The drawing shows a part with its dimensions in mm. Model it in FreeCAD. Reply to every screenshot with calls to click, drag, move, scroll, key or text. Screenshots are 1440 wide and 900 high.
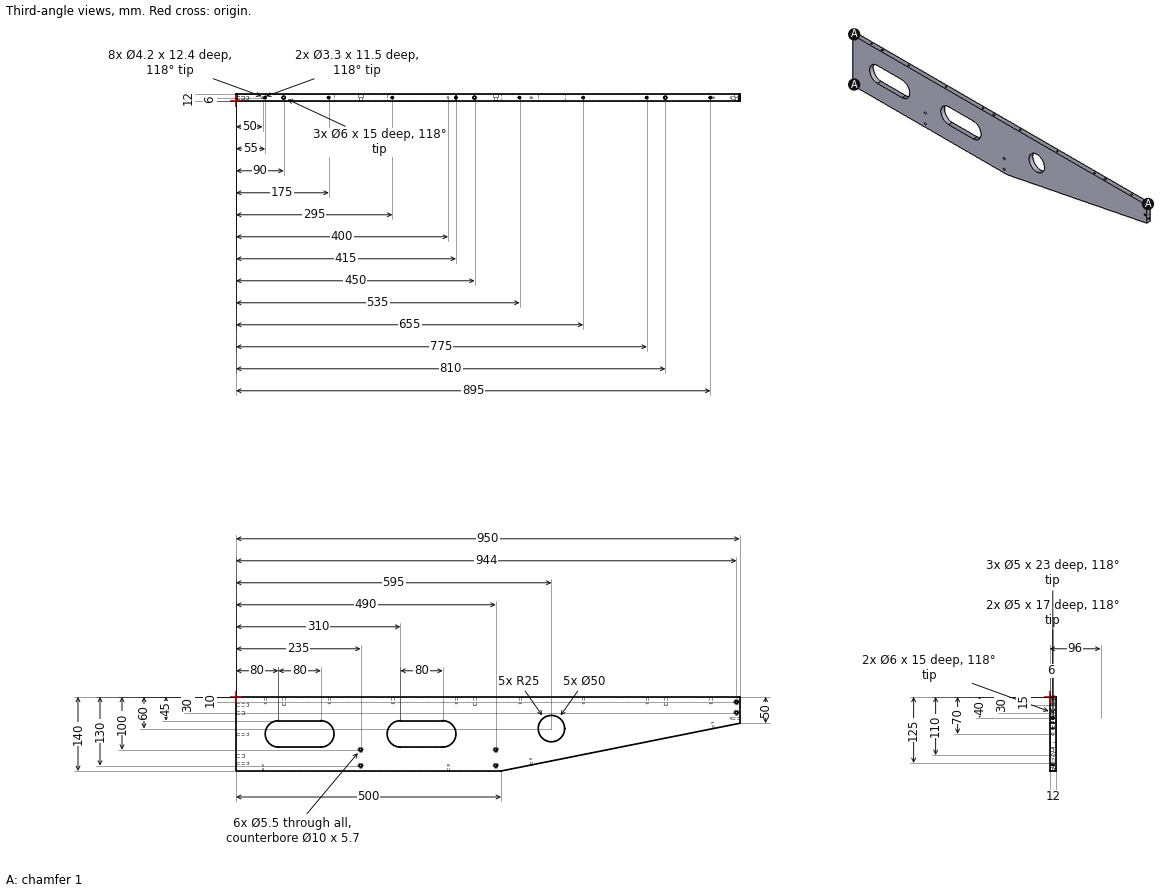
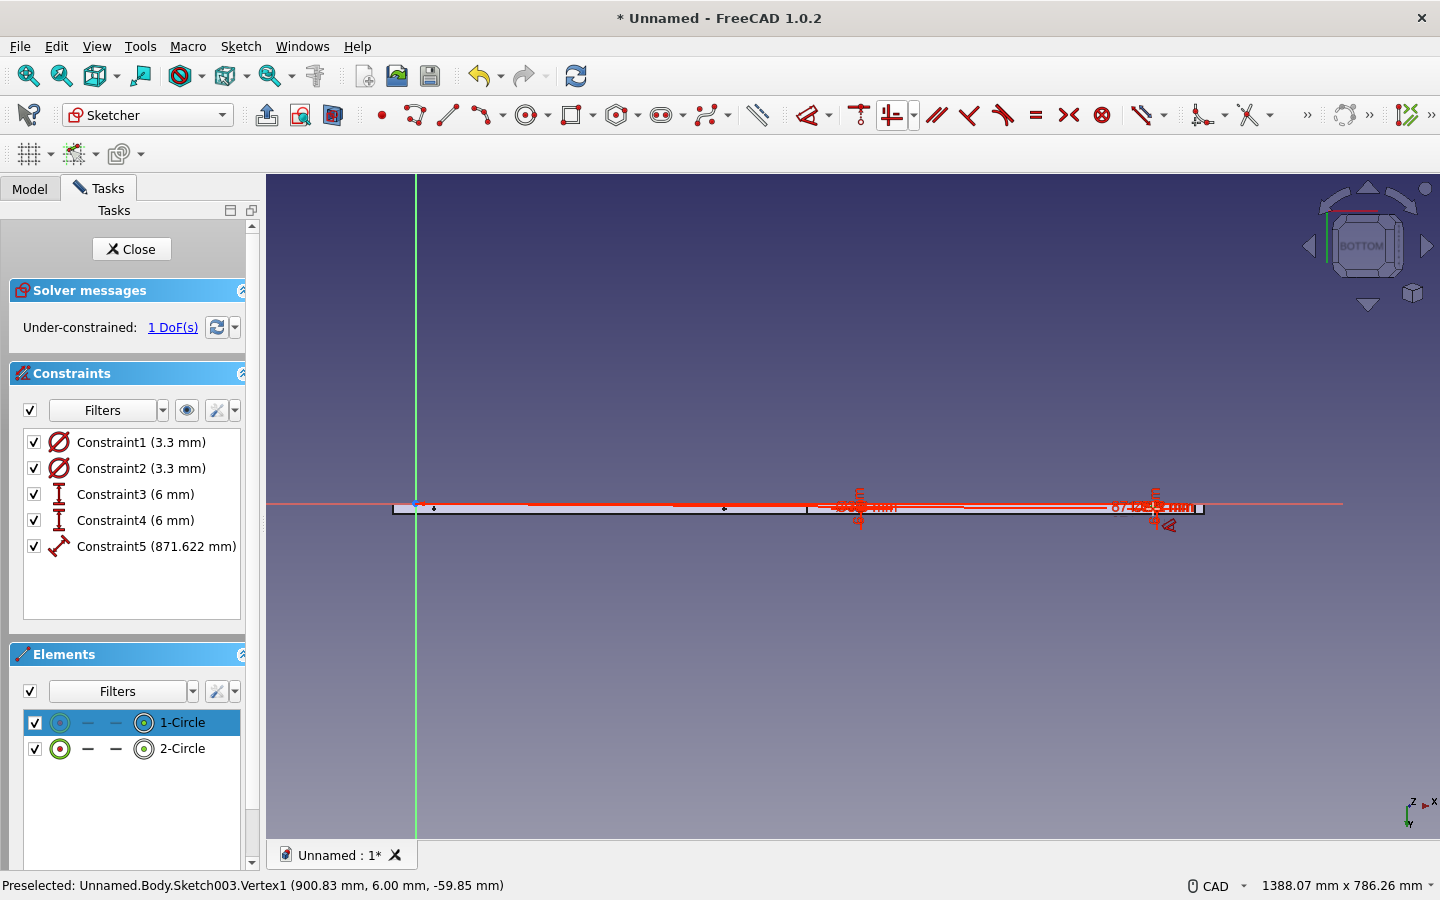
click(857, 509)
click(1005, 543)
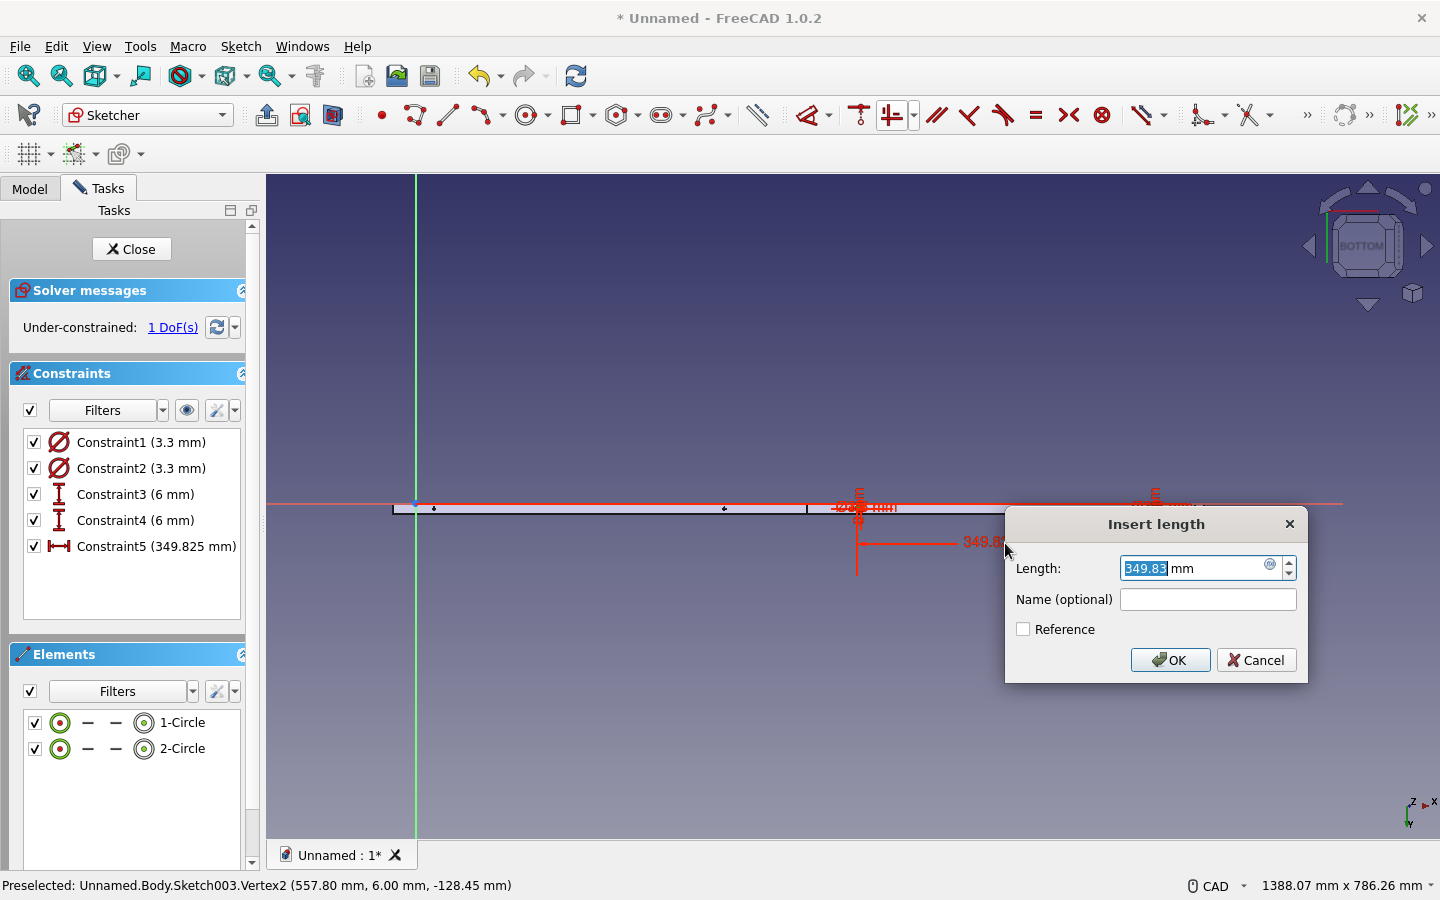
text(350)
key(Return)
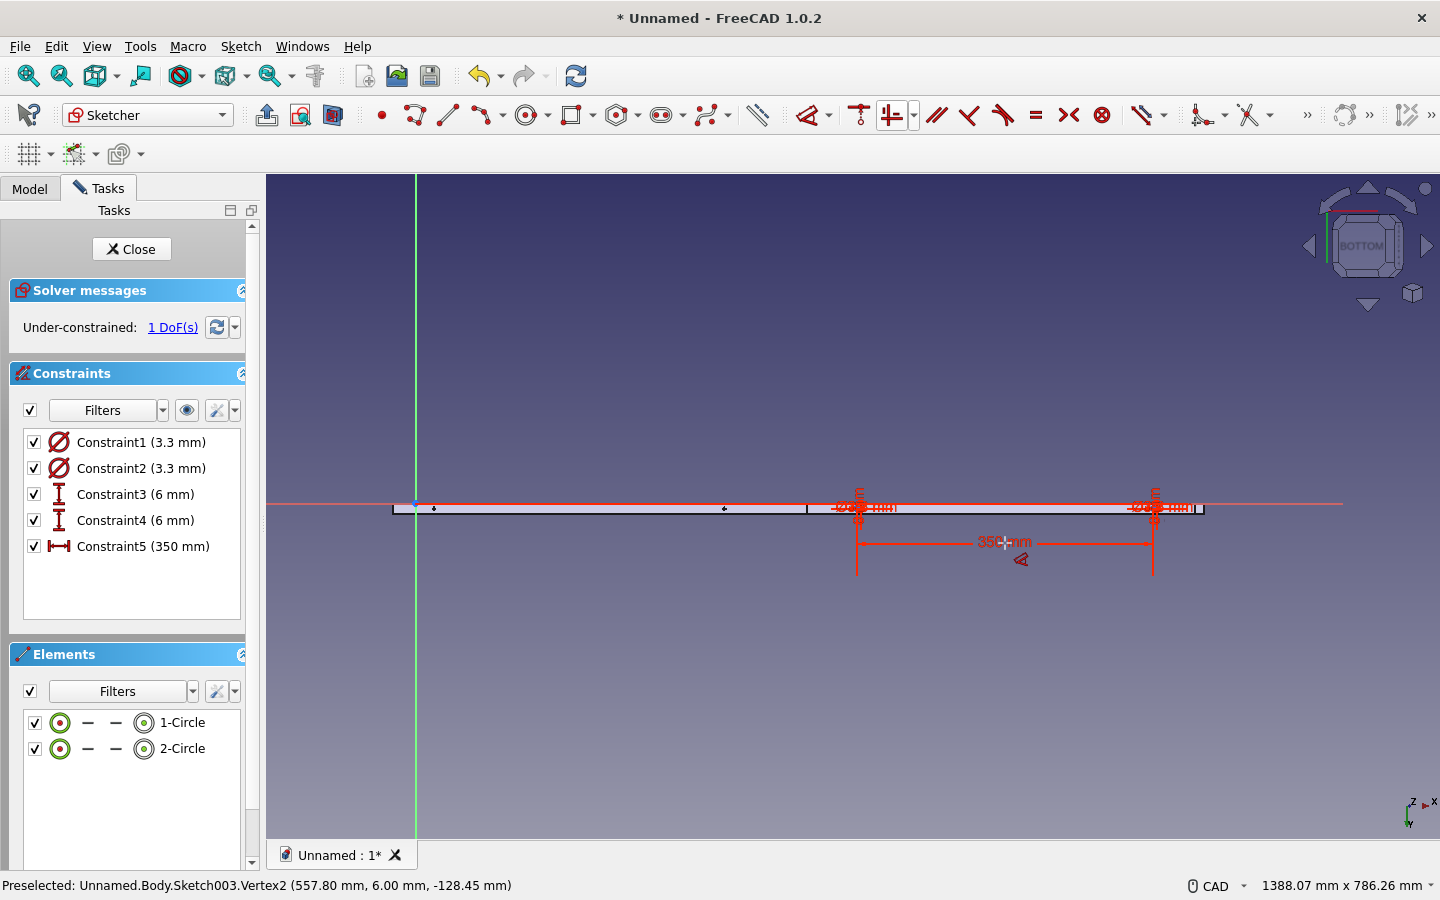
click(1153, 509)
click(784, 470)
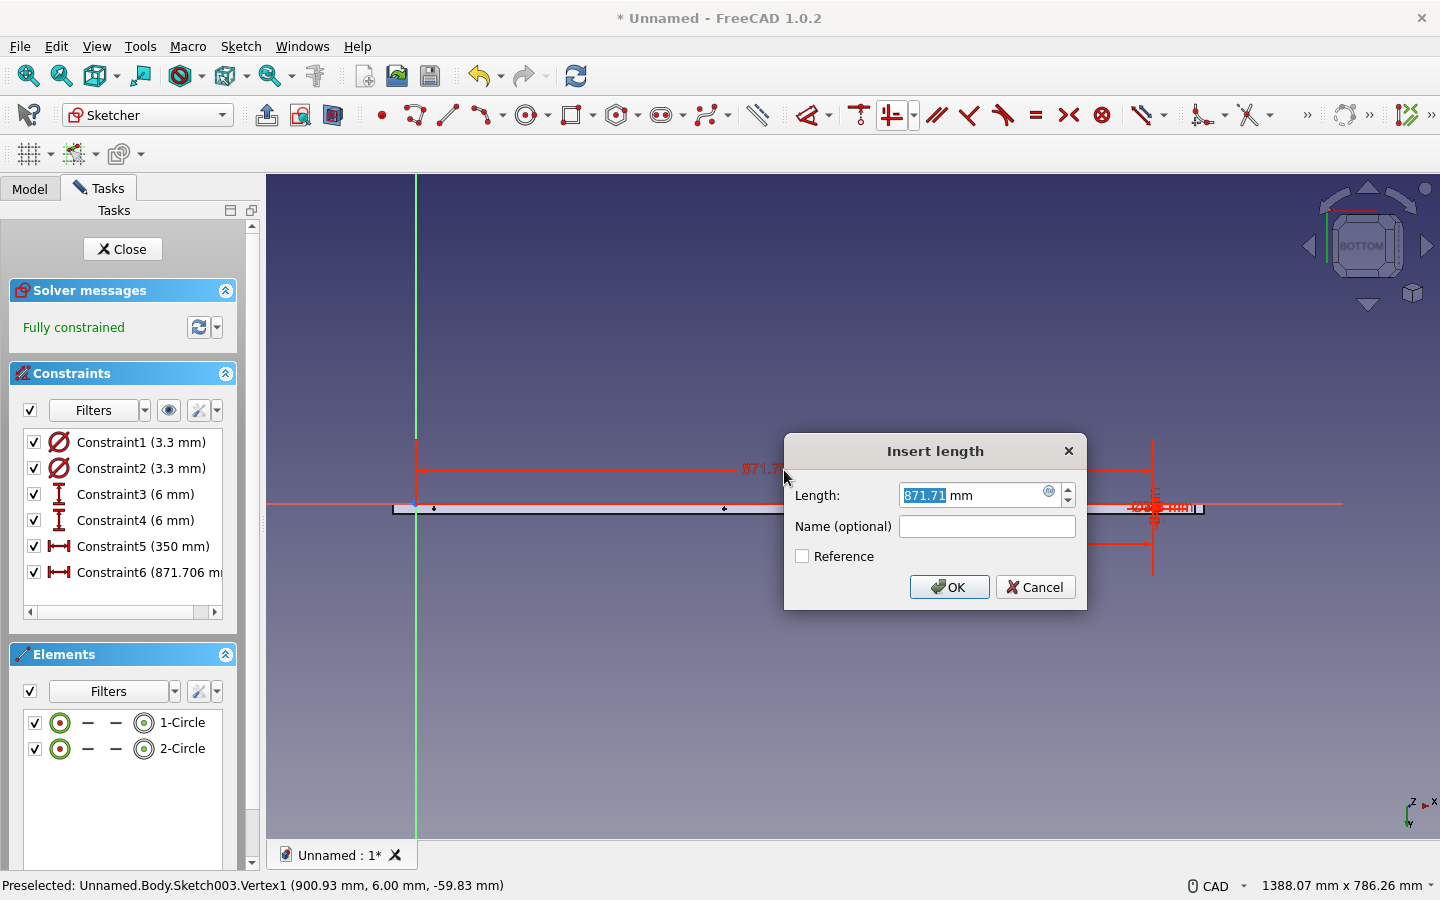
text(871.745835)
key(Return)
key(Escape)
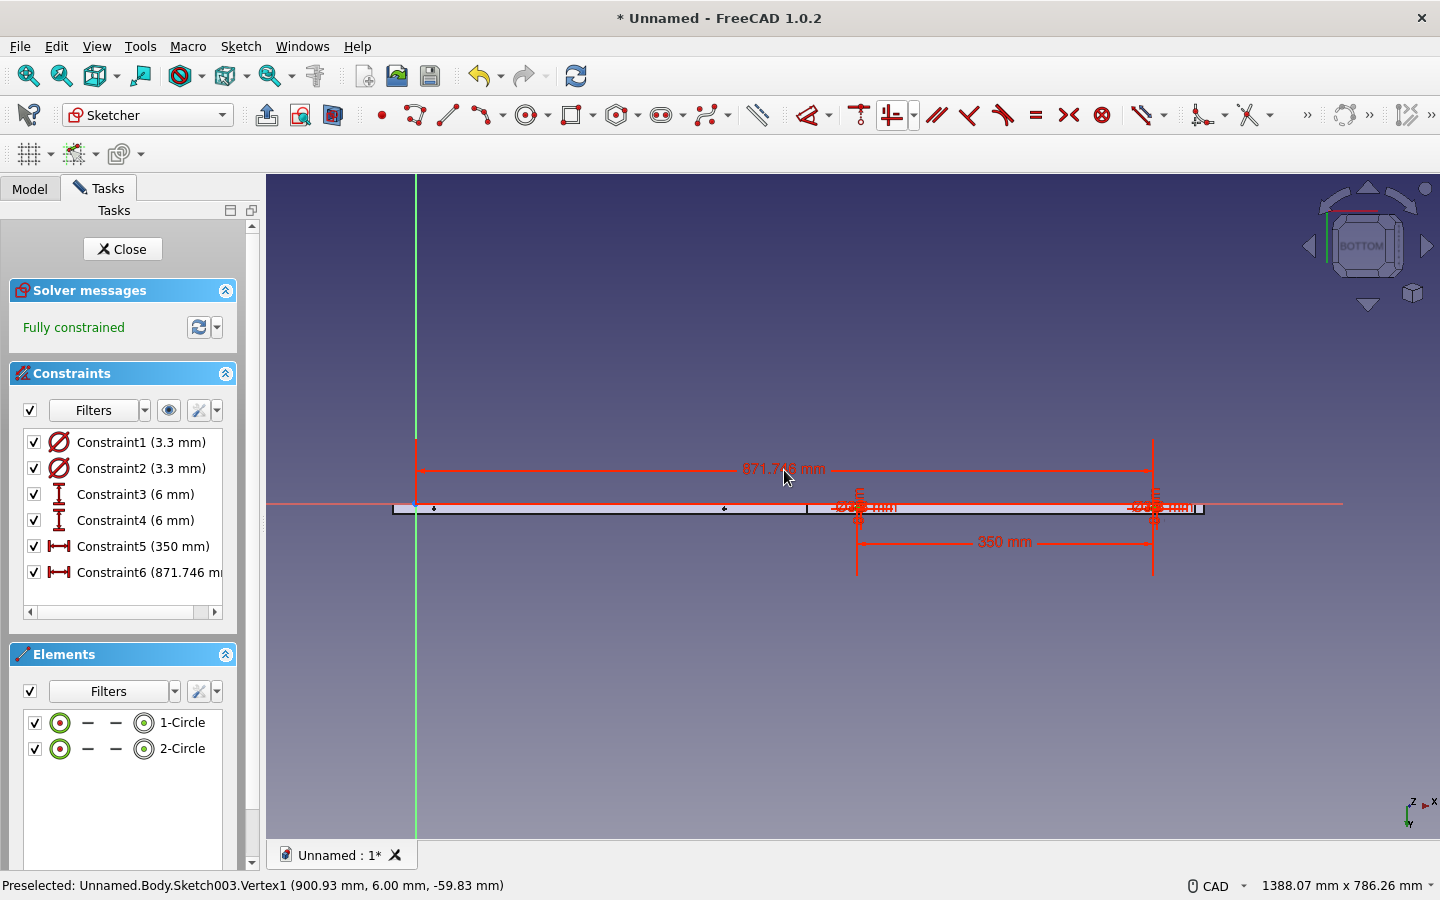
click(123, 249)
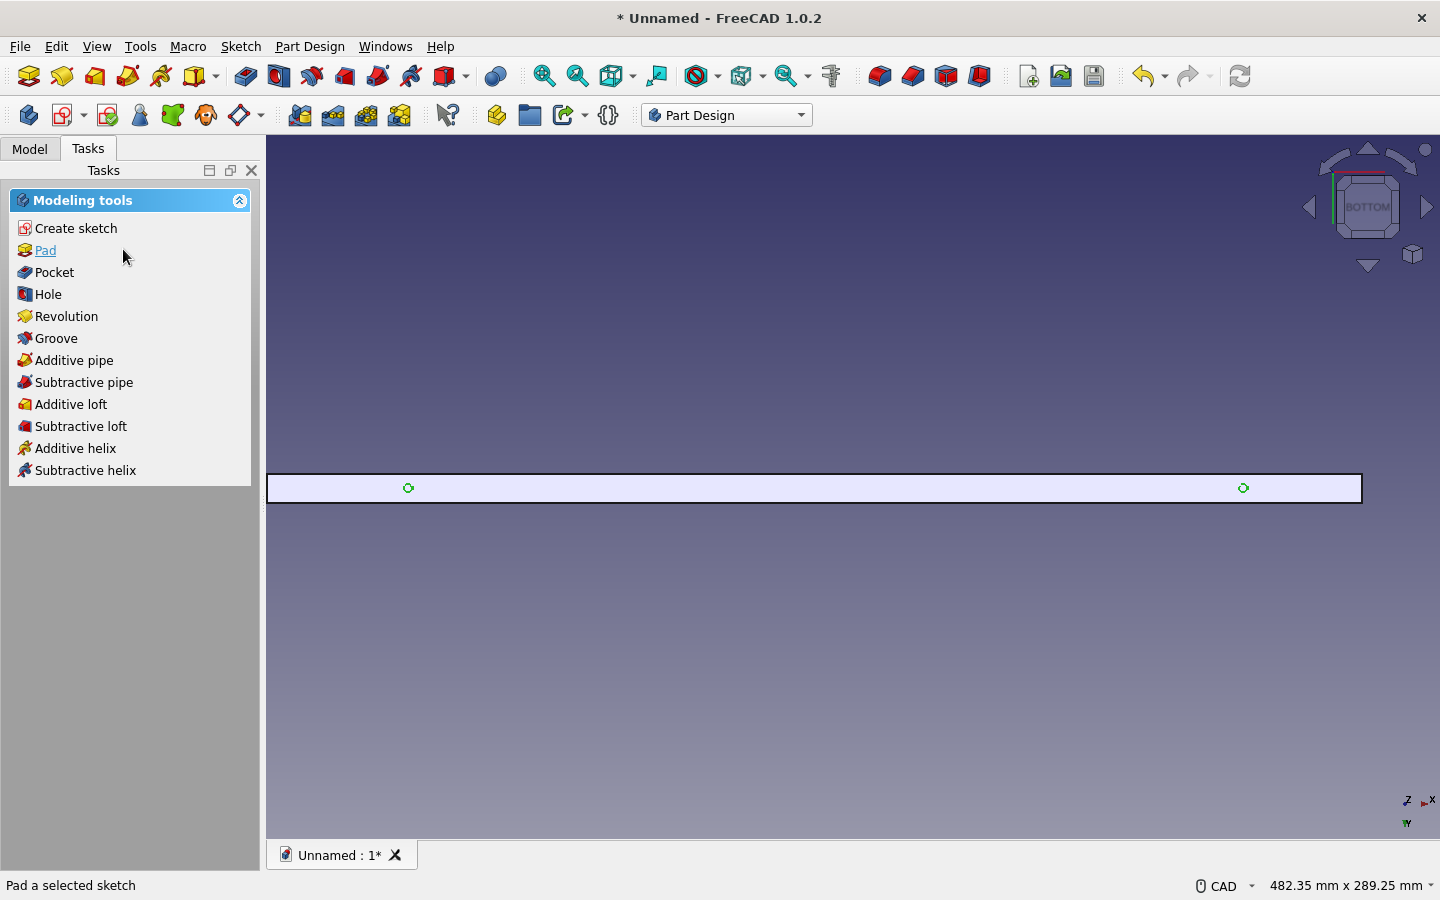
click(279, 76)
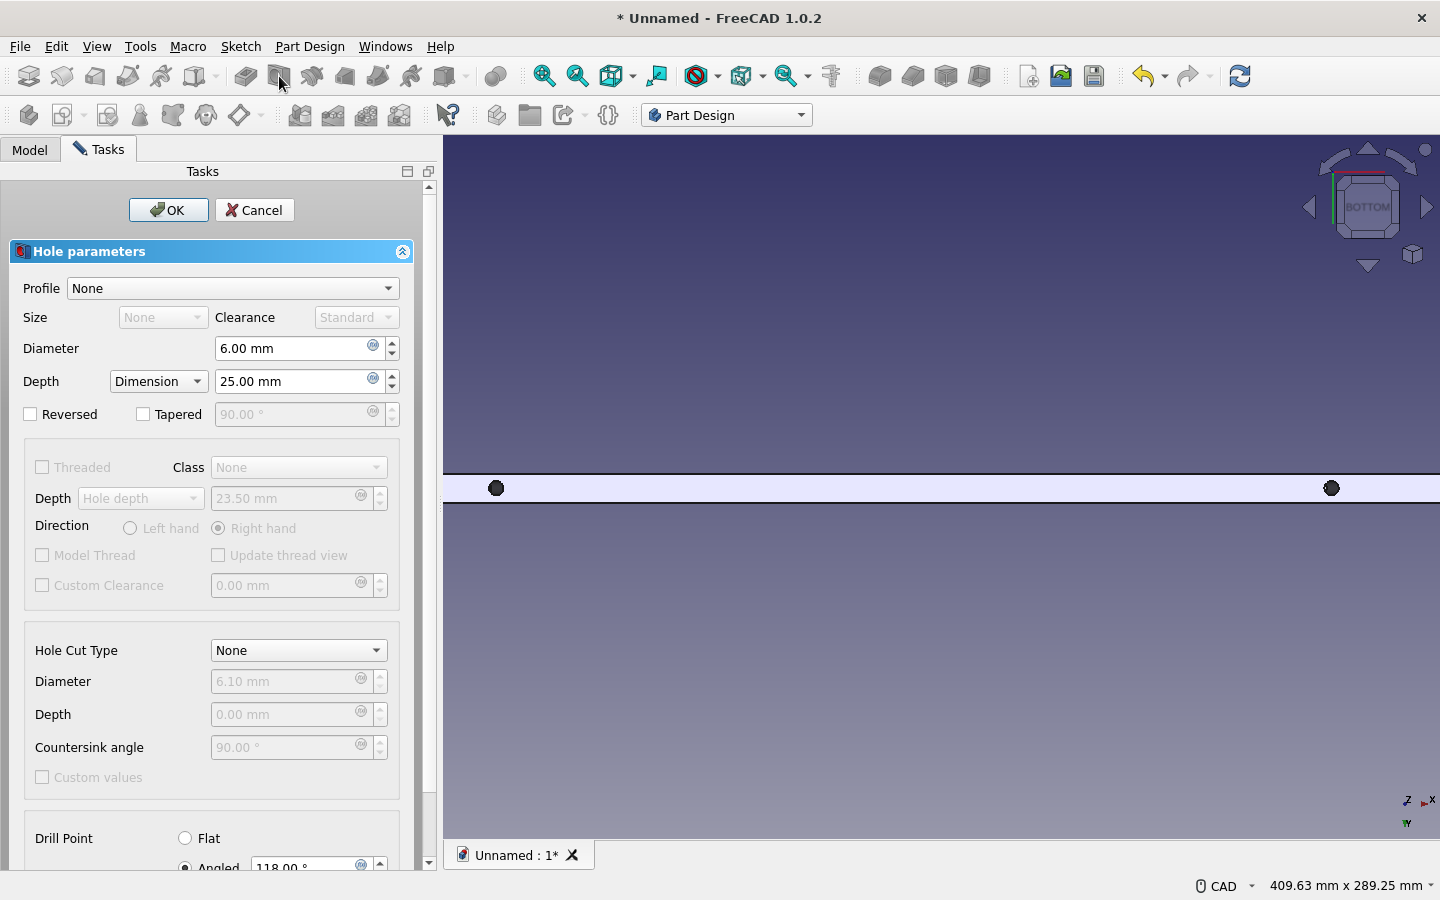
triple_click(300, 348)